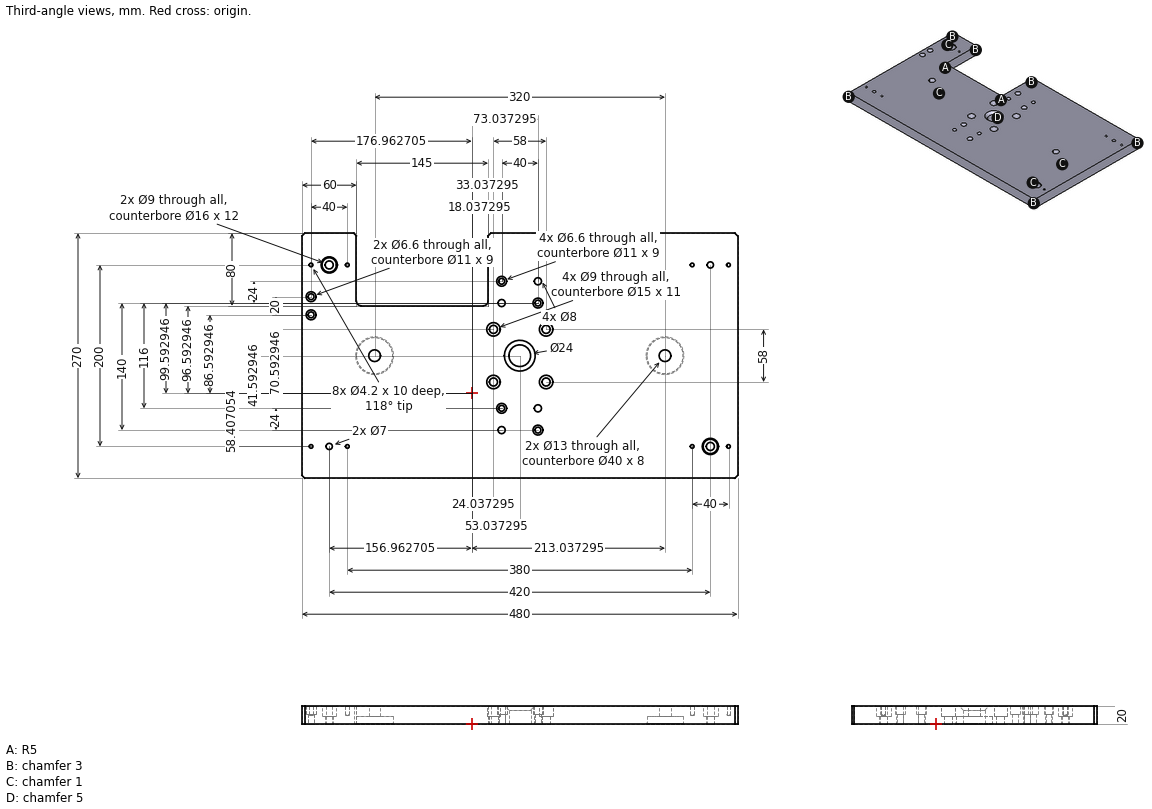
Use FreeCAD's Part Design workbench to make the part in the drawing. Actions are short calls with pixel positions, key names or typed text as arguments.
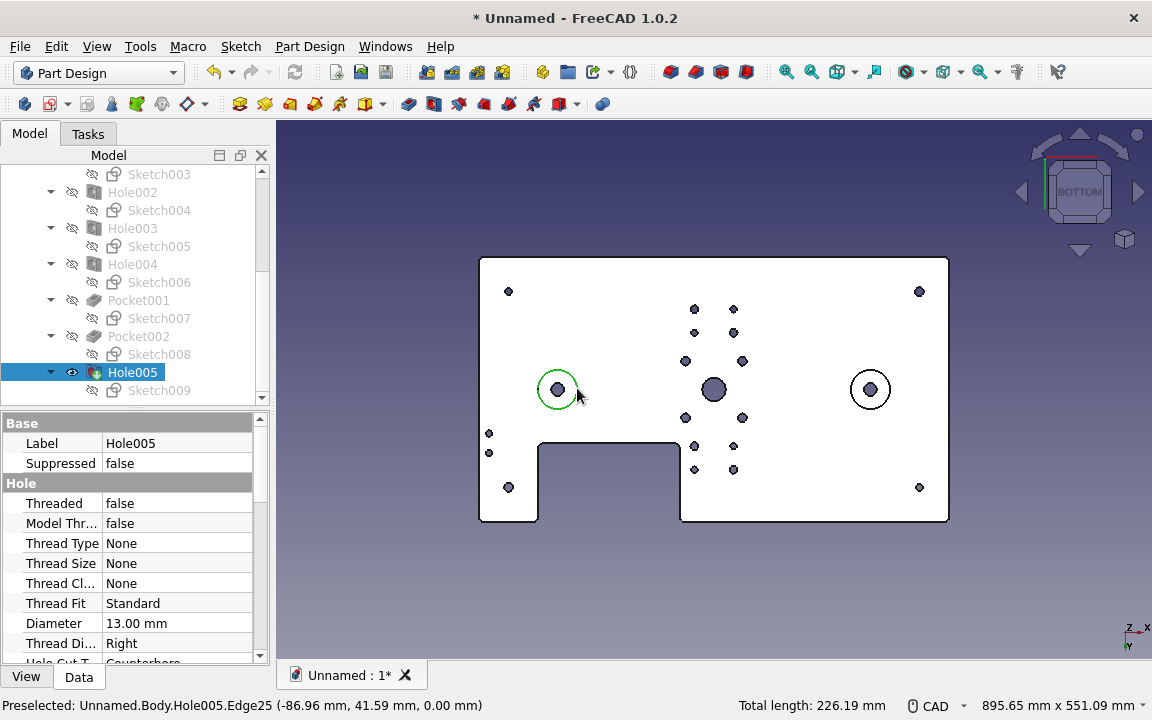
click(890, 388, ctrl)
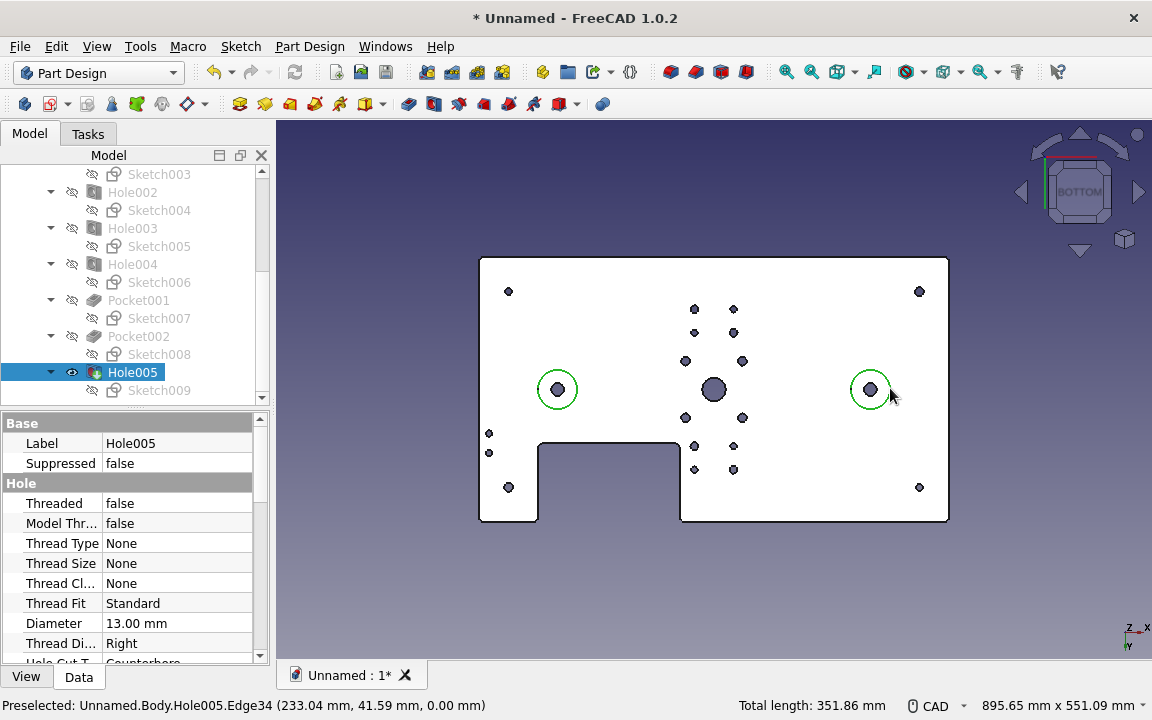
click(696, 72)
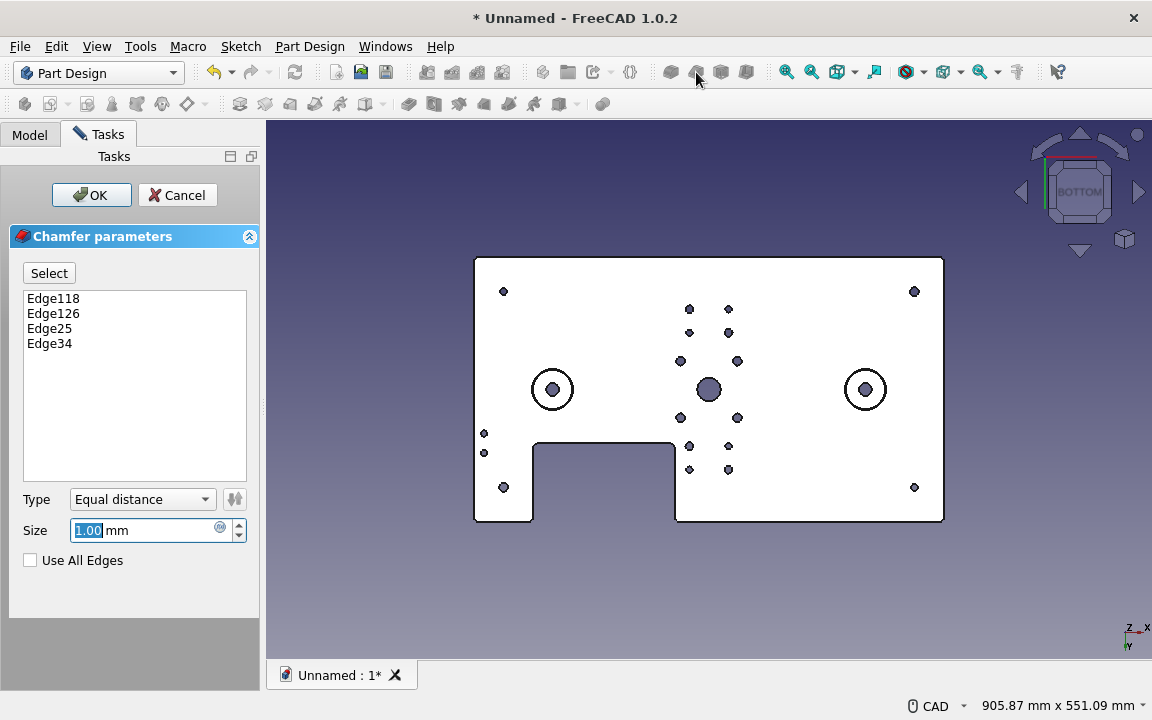
text(1)
key(Tab)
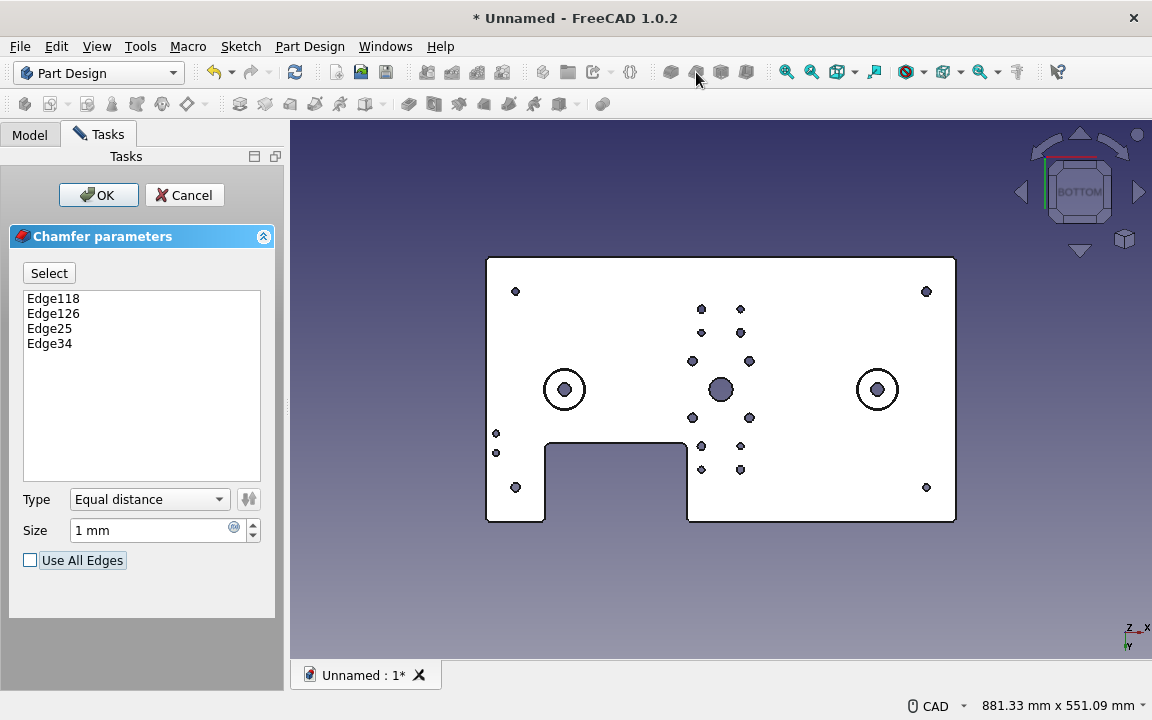
click(99, 195)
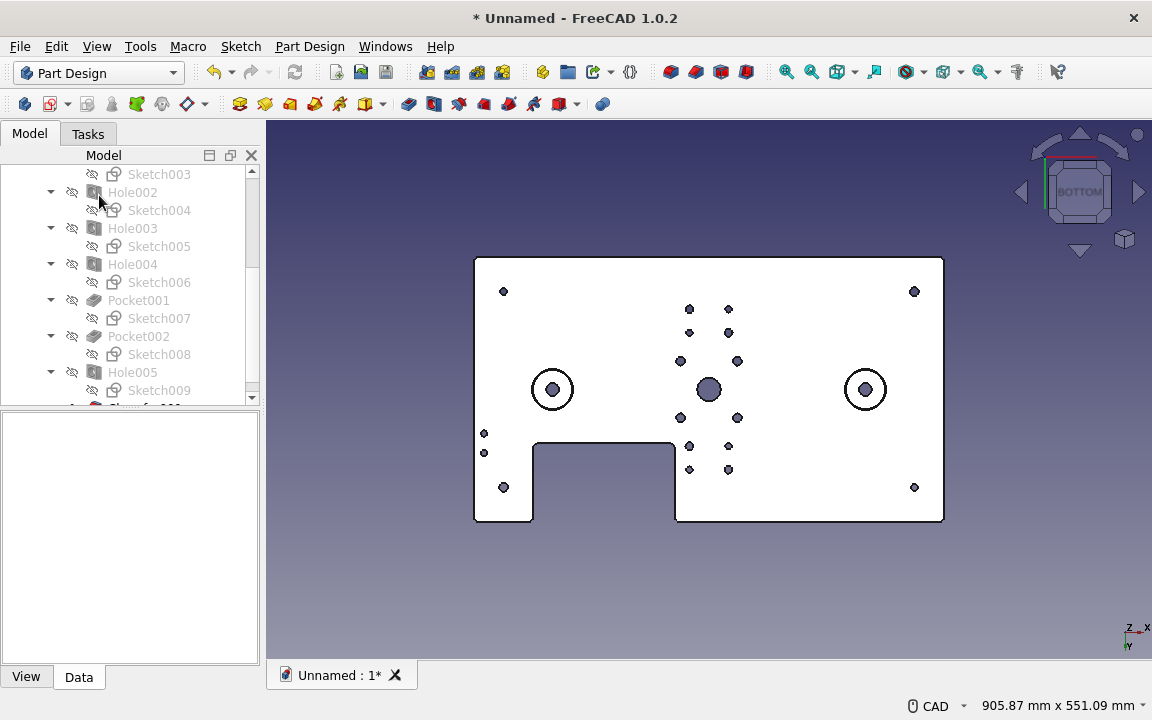
key(0)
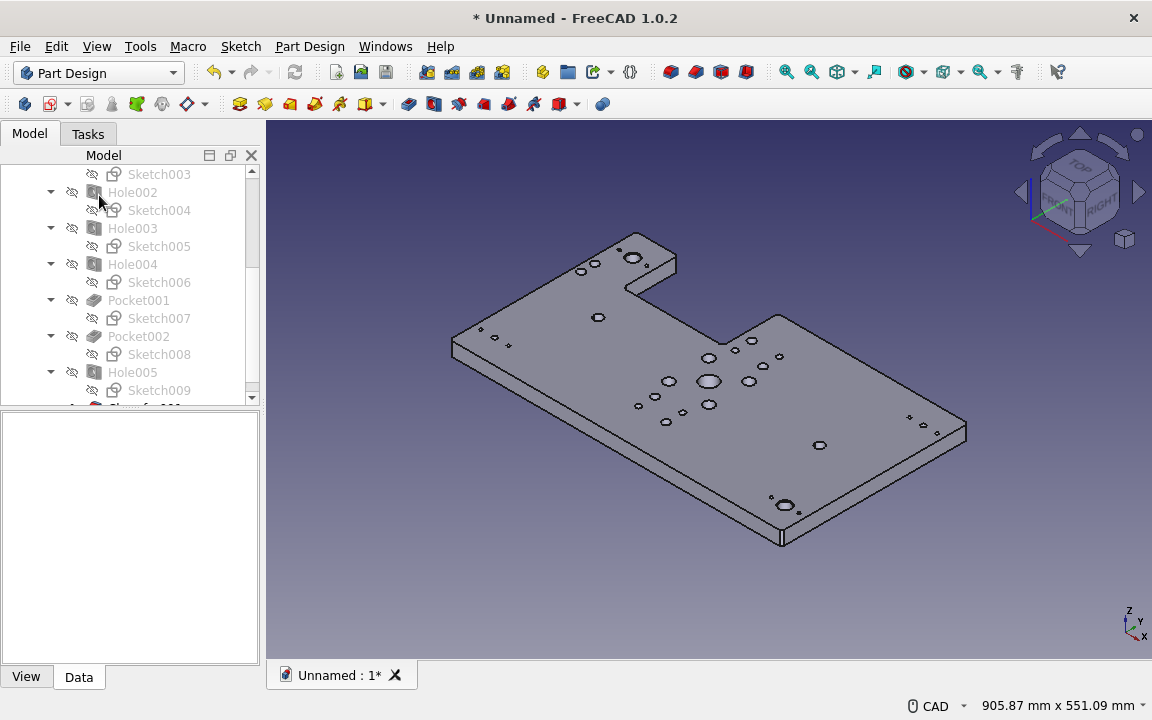
click(701, 376)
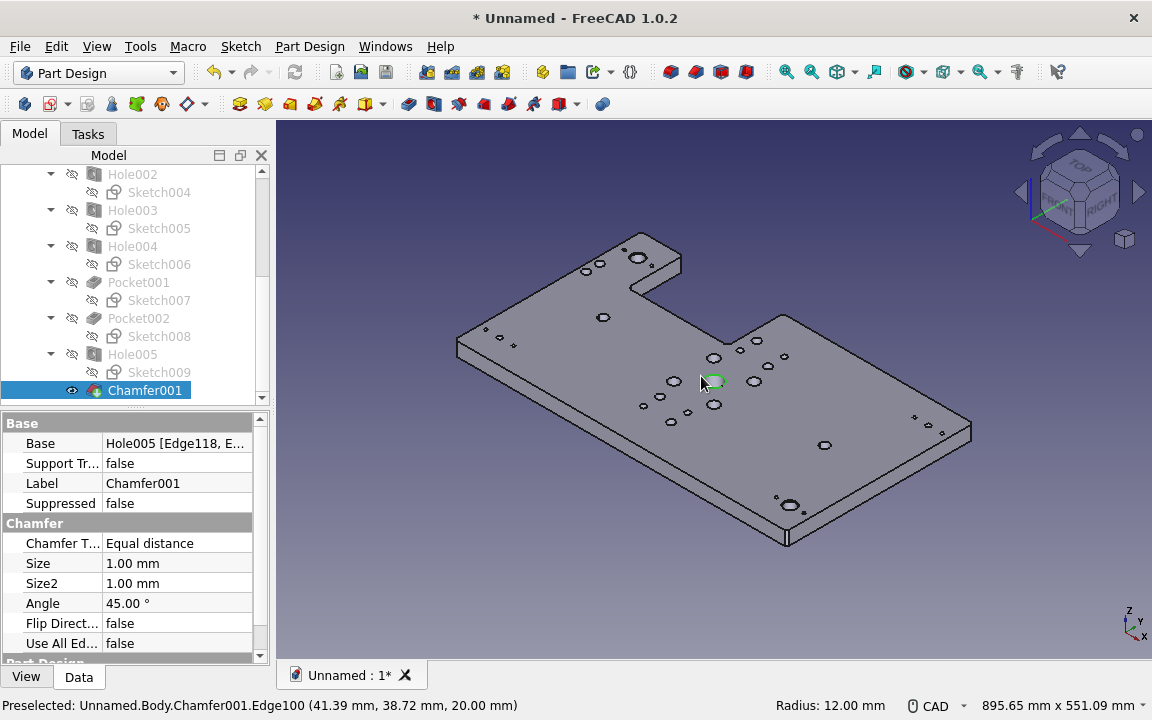
click(696, 72)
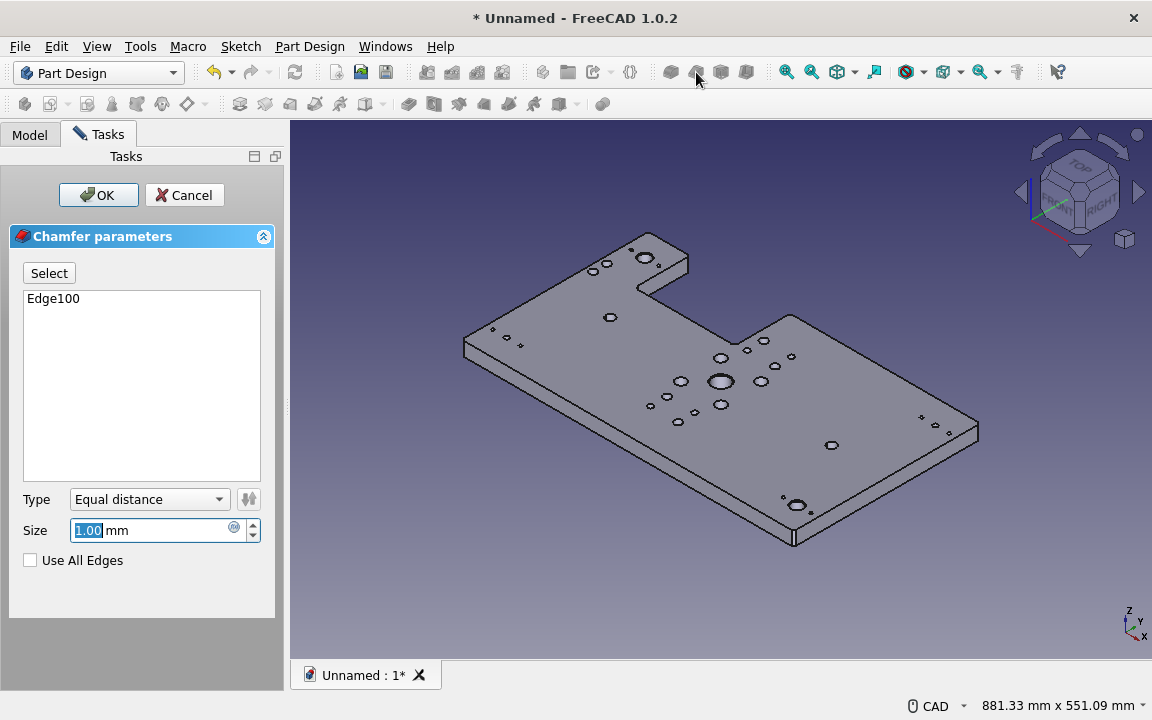
text(5)
key(Tab)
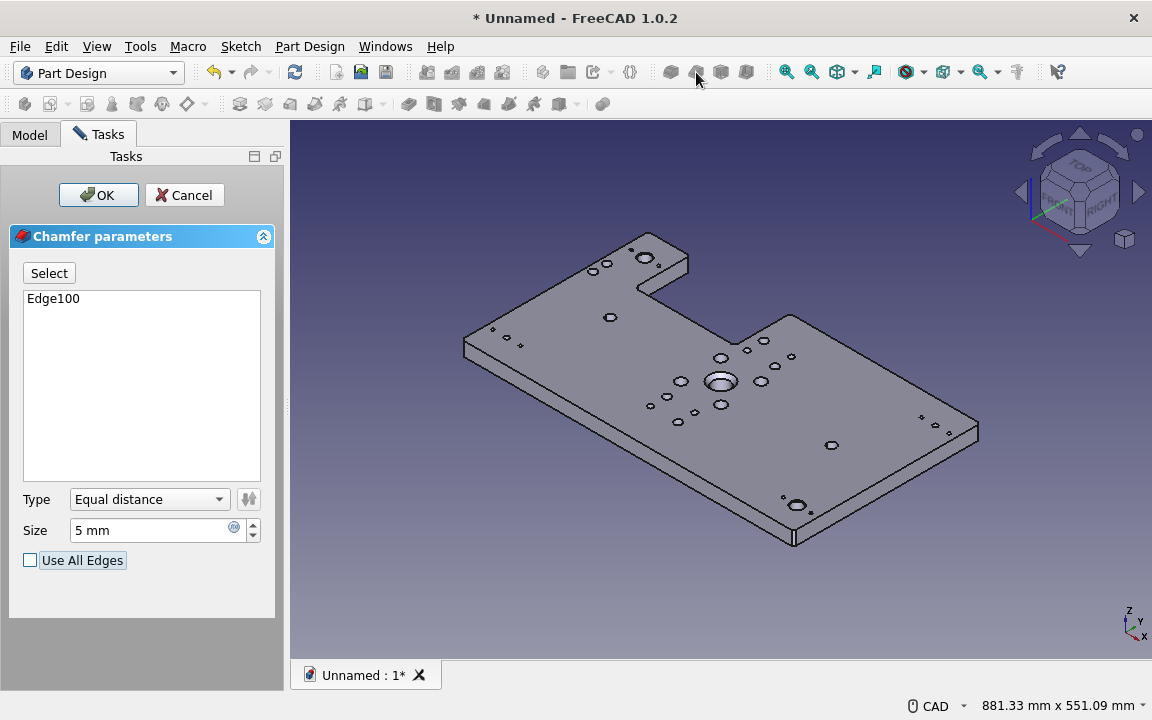
click(99, 195)